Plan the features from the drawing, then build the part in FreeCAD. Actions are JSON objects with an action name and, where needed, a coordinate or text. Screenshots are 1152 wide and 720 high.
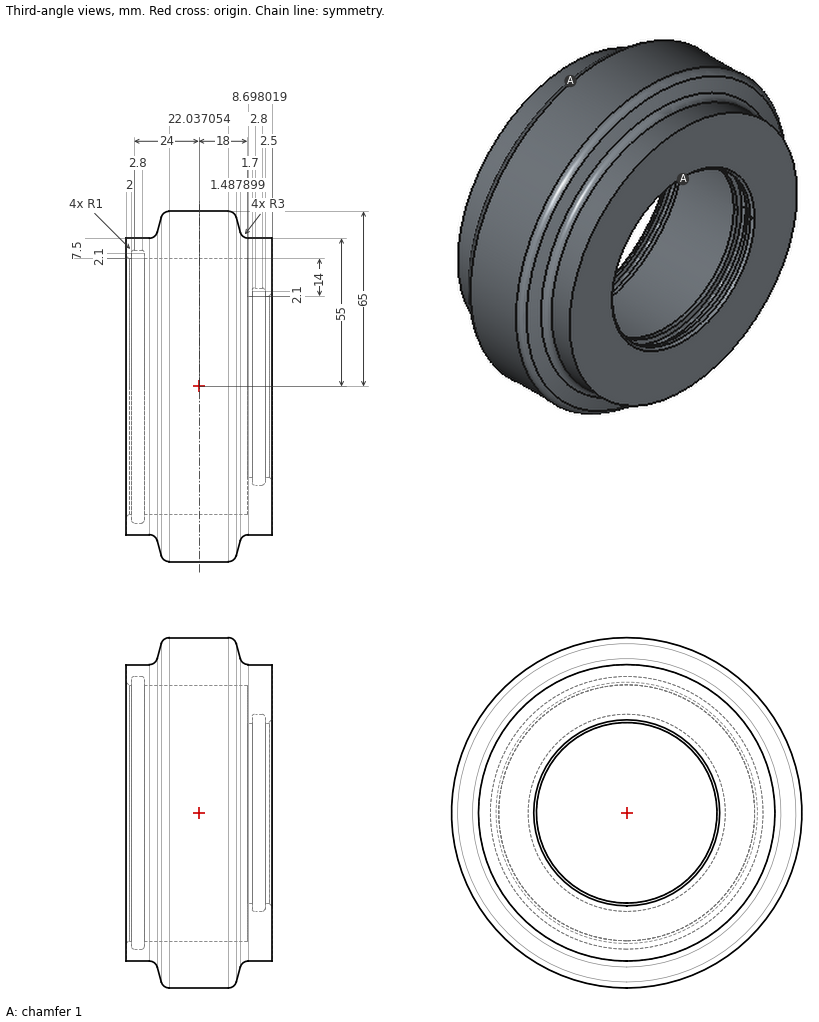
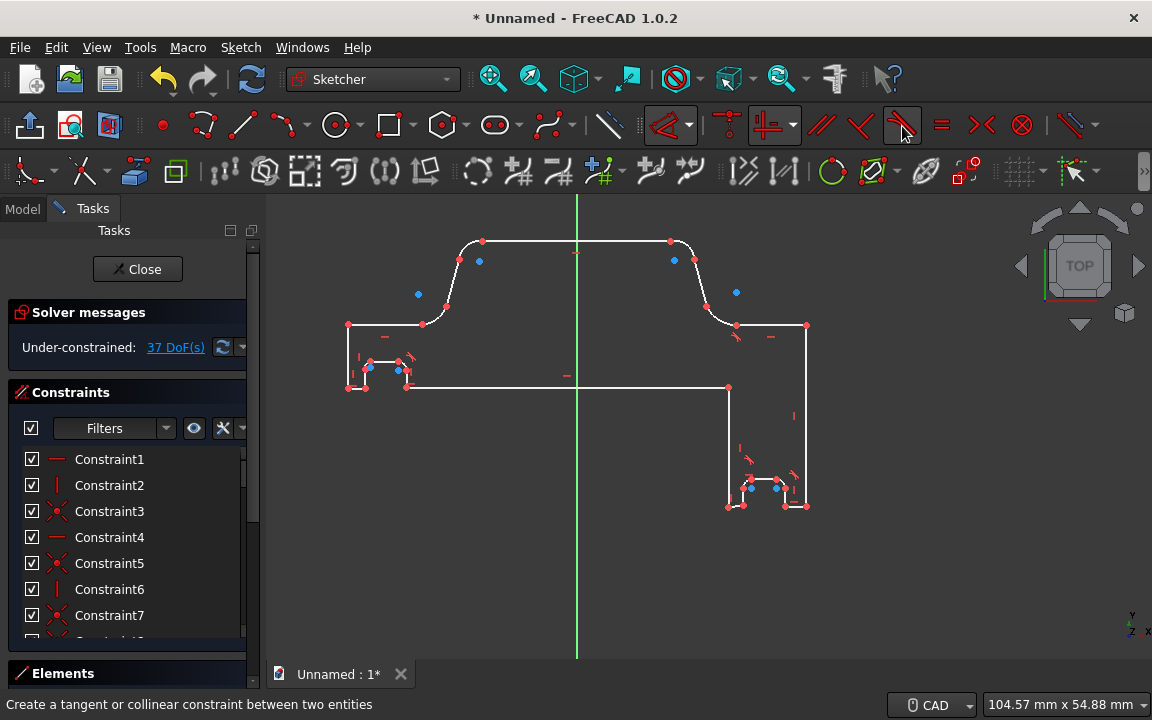
{"action": "left_click", "coordinate": [703, 292]}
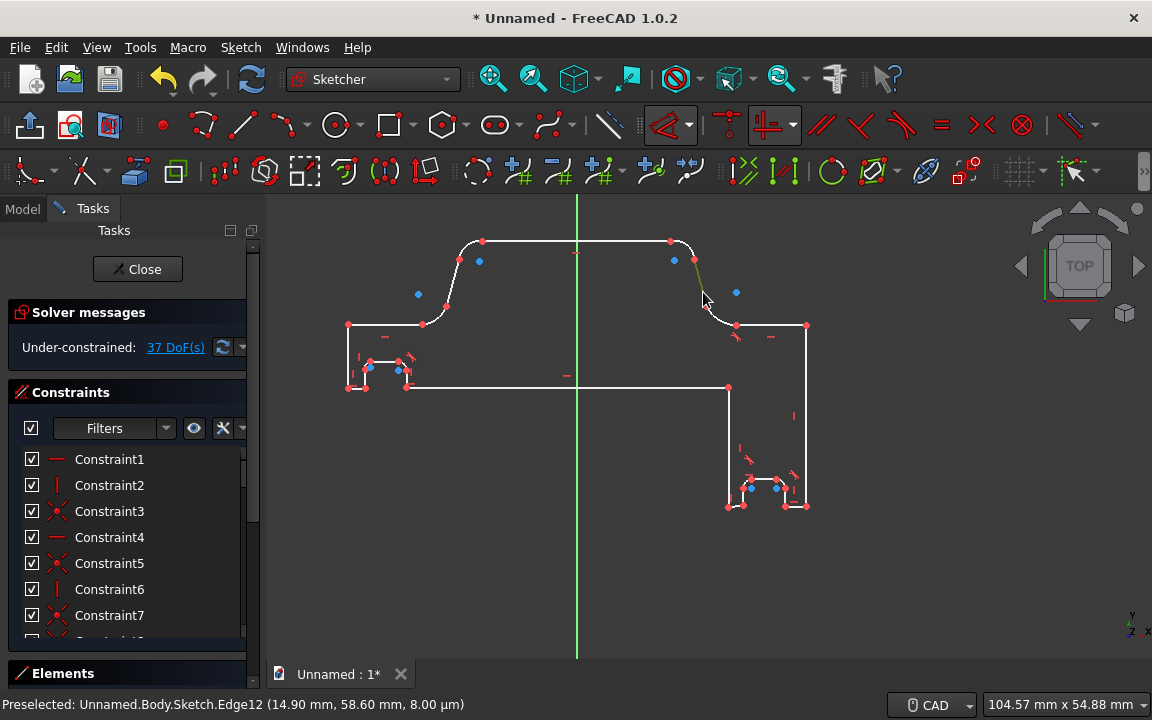
{"action": "scroll", "coordinate": [713, 316], "scroll_direction": "up", "scroll_amount": 2}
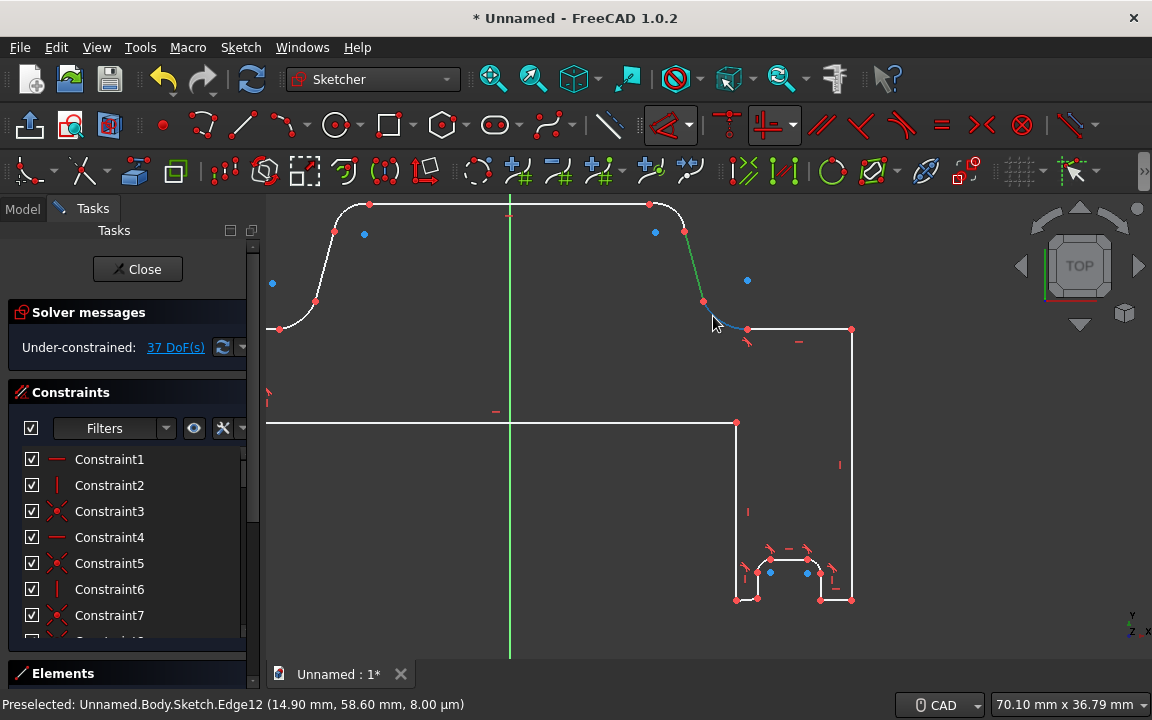
{"action": "left_click", "coordinate": [713, 315]}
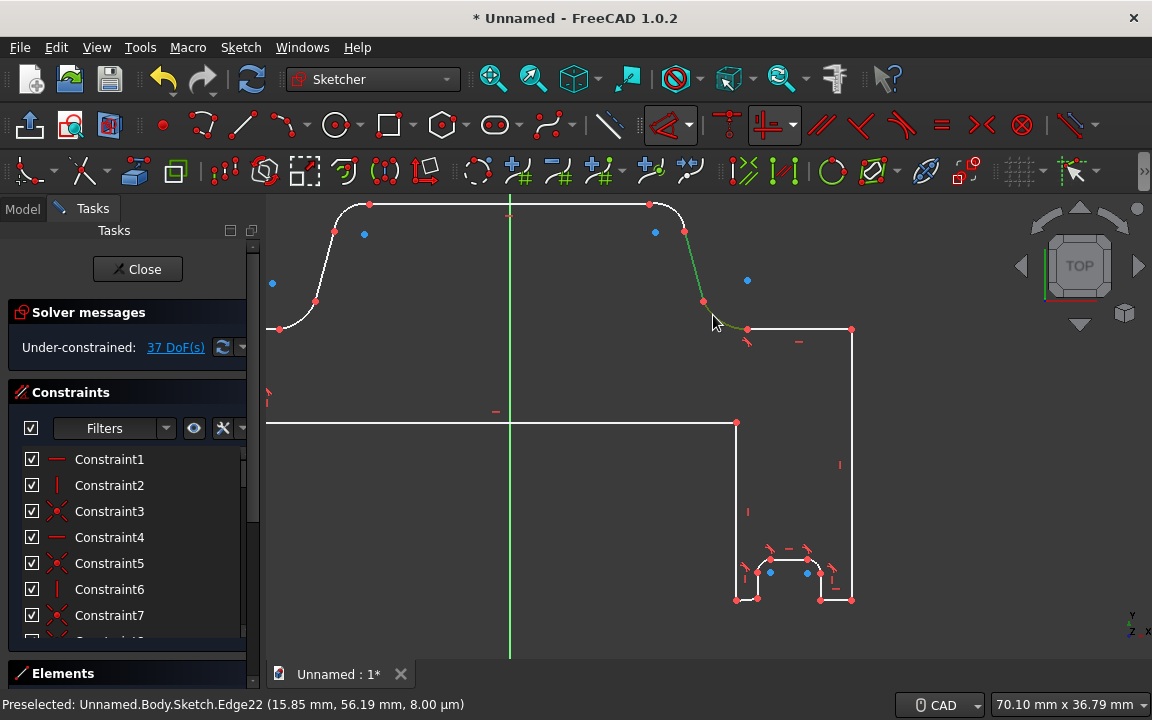
{"action": "key", "text": "t"}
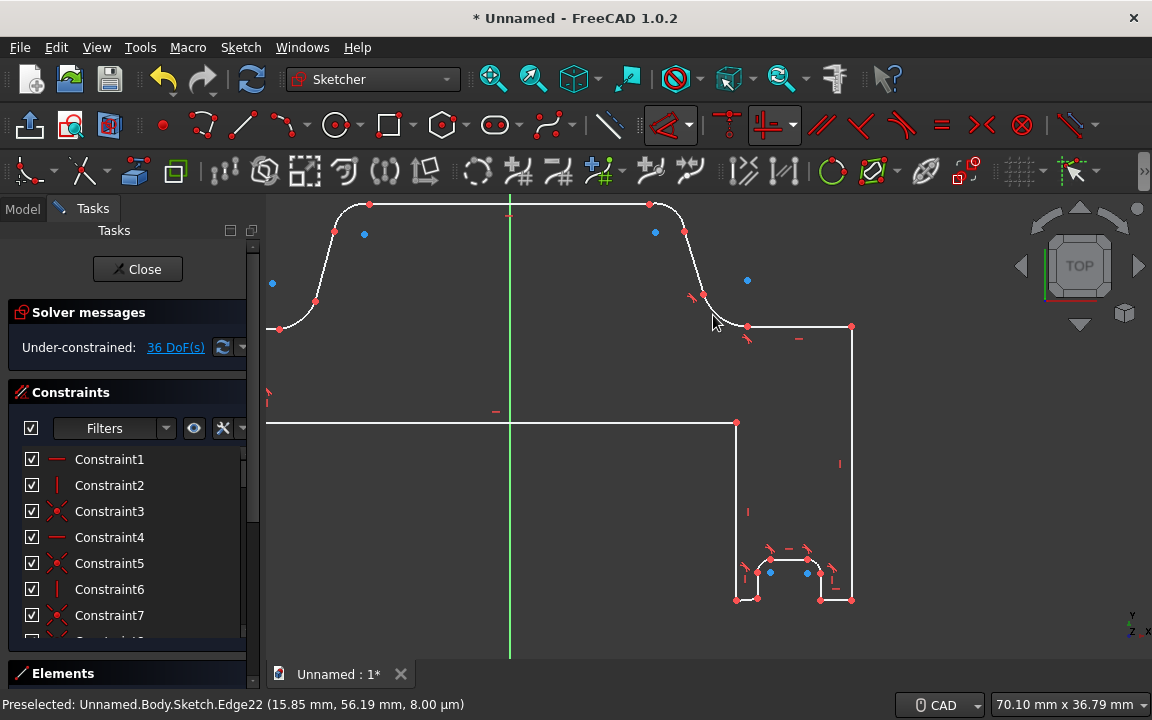
{"action": "left_click", "coordinate": [698, 275]}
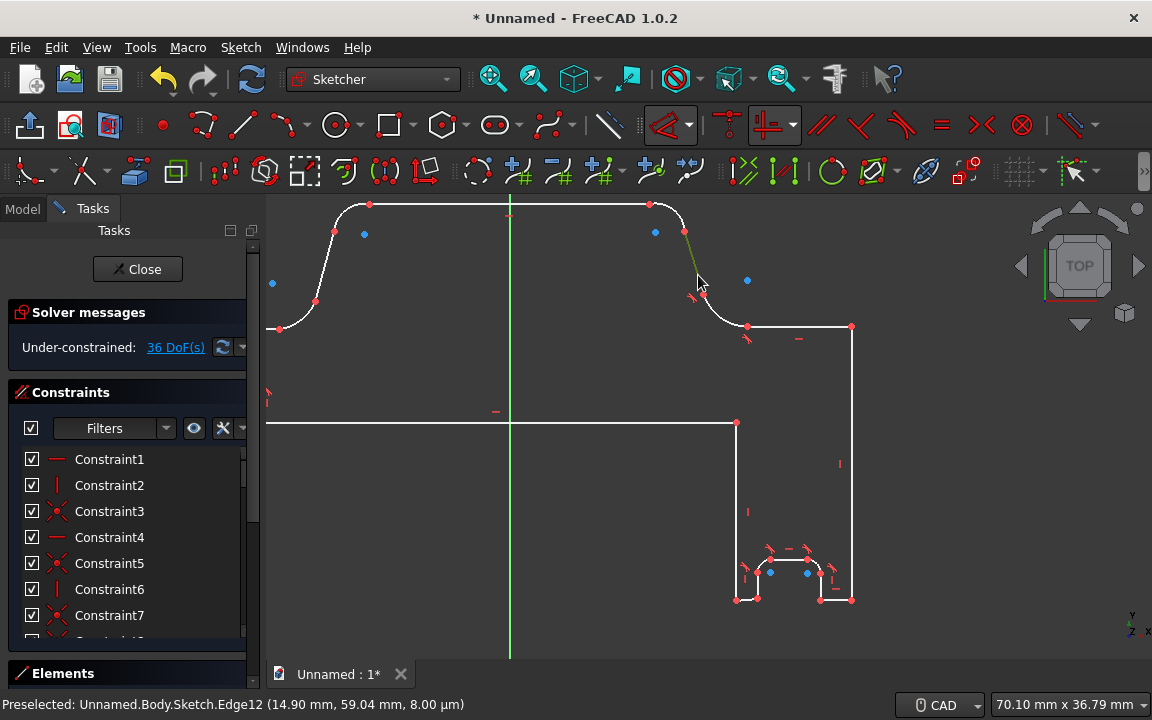
{"action": "scroll", "coordinate": [716, 319], "scroll_direction": "down", "scroll_amount": 5}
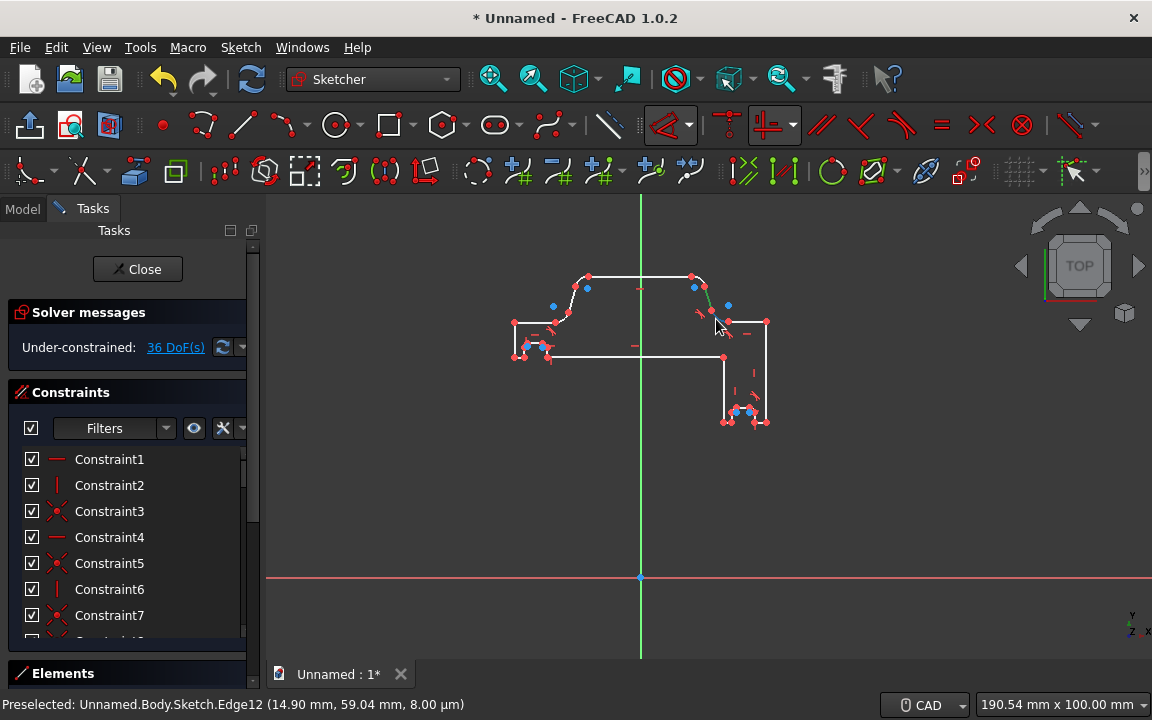
{"action": "scroll", "coordinate": [703, 282], "scroll_direction": "up", "scroll_amount": 5}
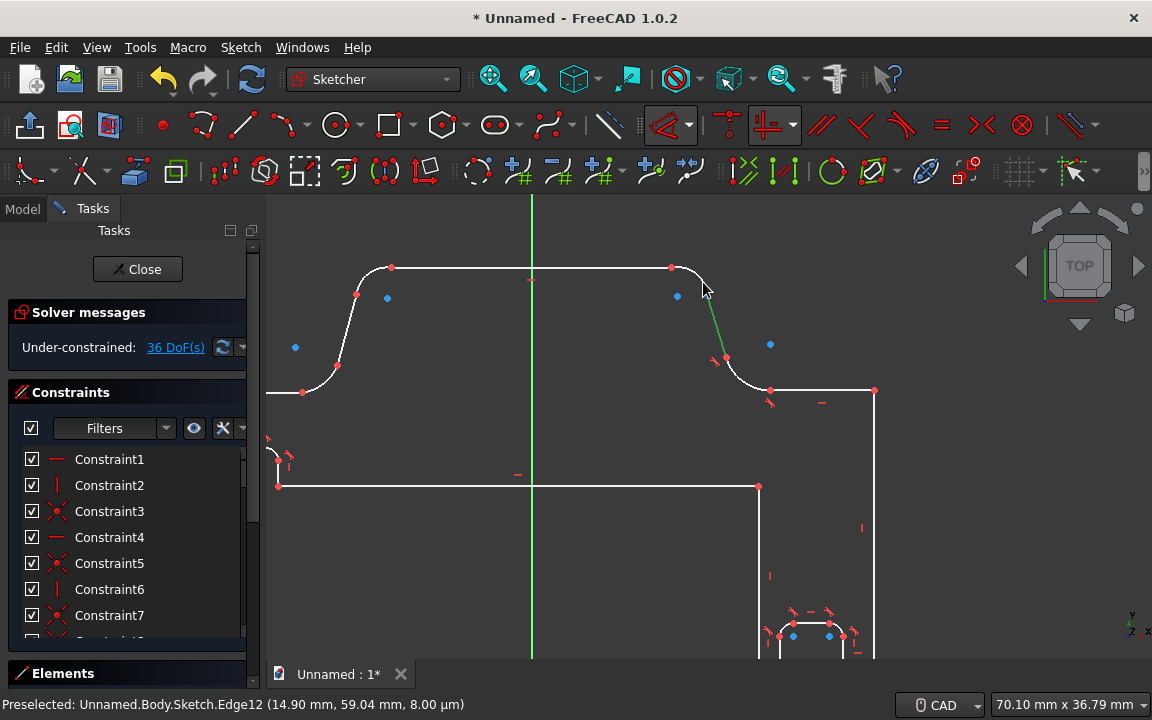
{"action": "left_click", "coordinate": [702, 281]}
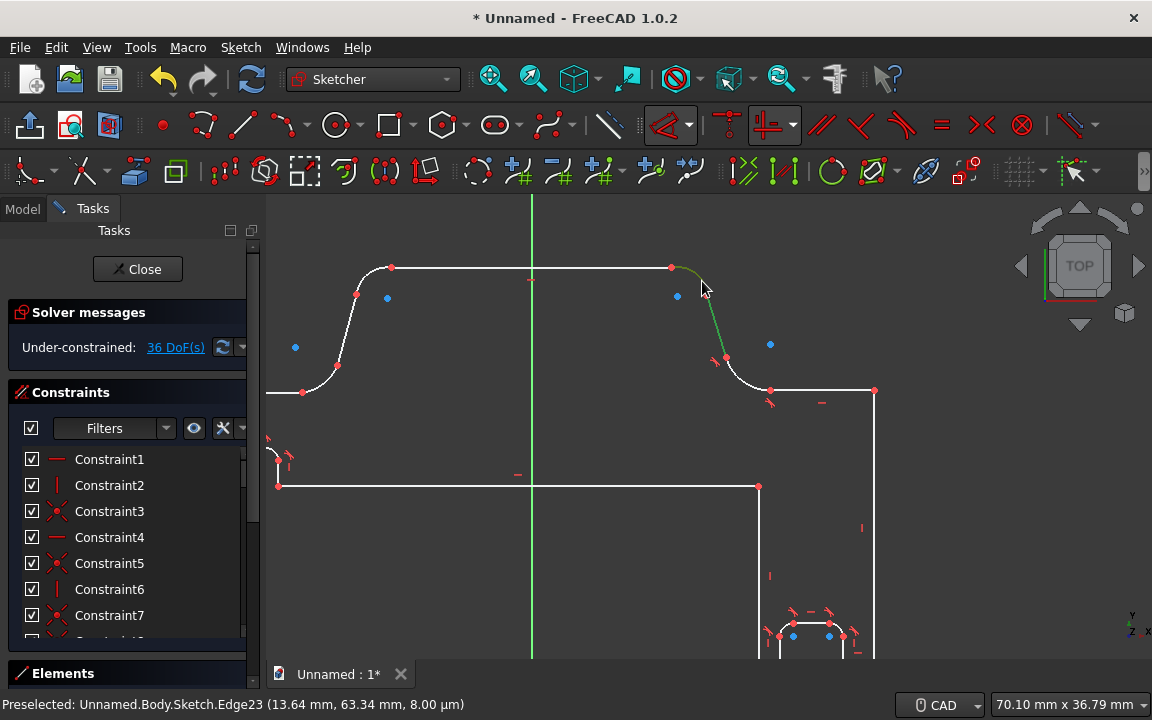
{"action": "key", "text": "t"}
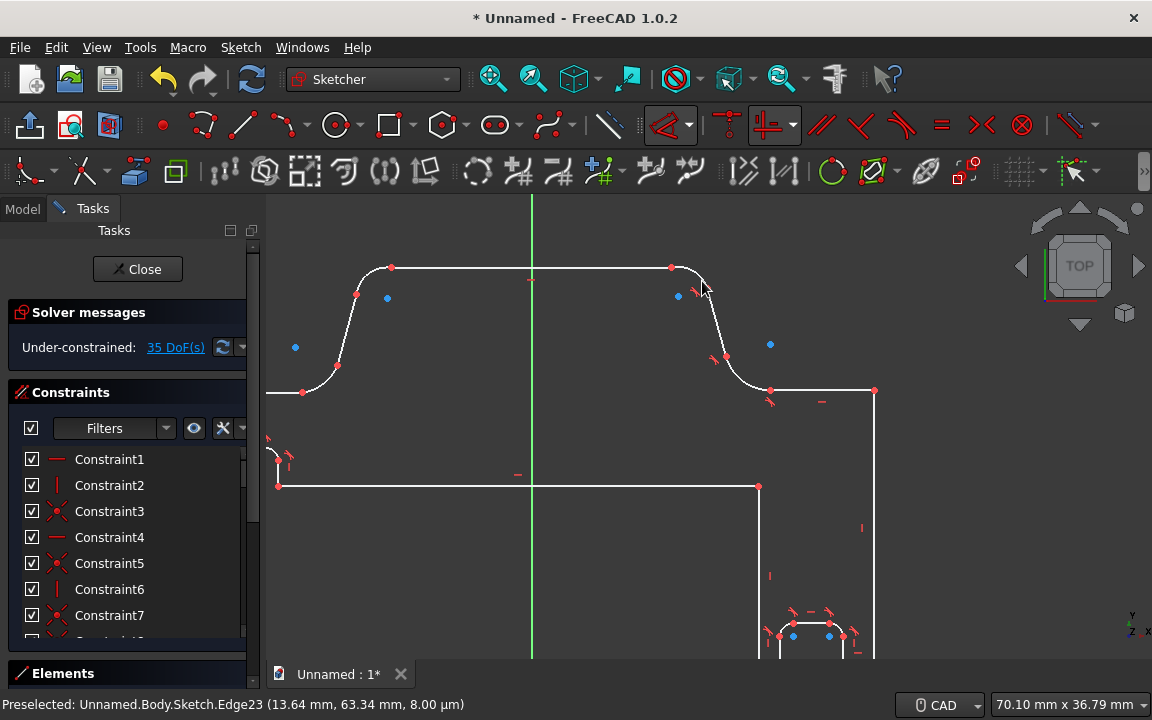
{"action": "left_click", "coordinate": [588, 268]}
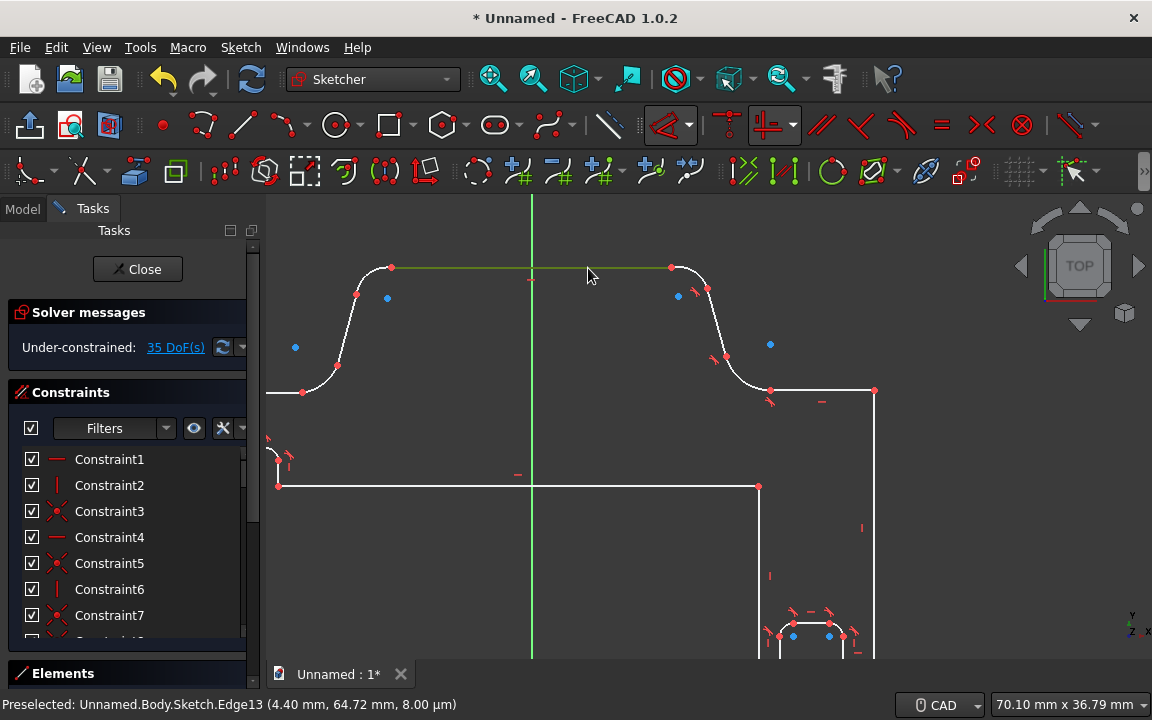
{"action": "left_click", "coordinate": [701, 277]}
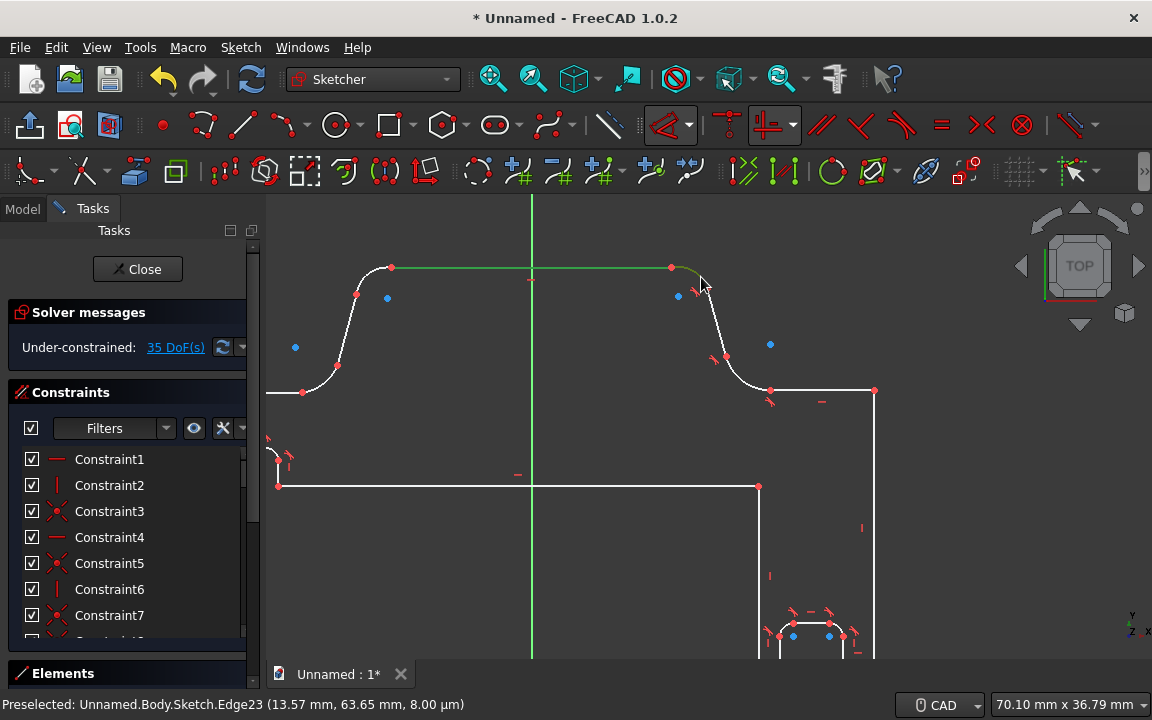
{"action": "left_click", "coordinate": [902, 126]}